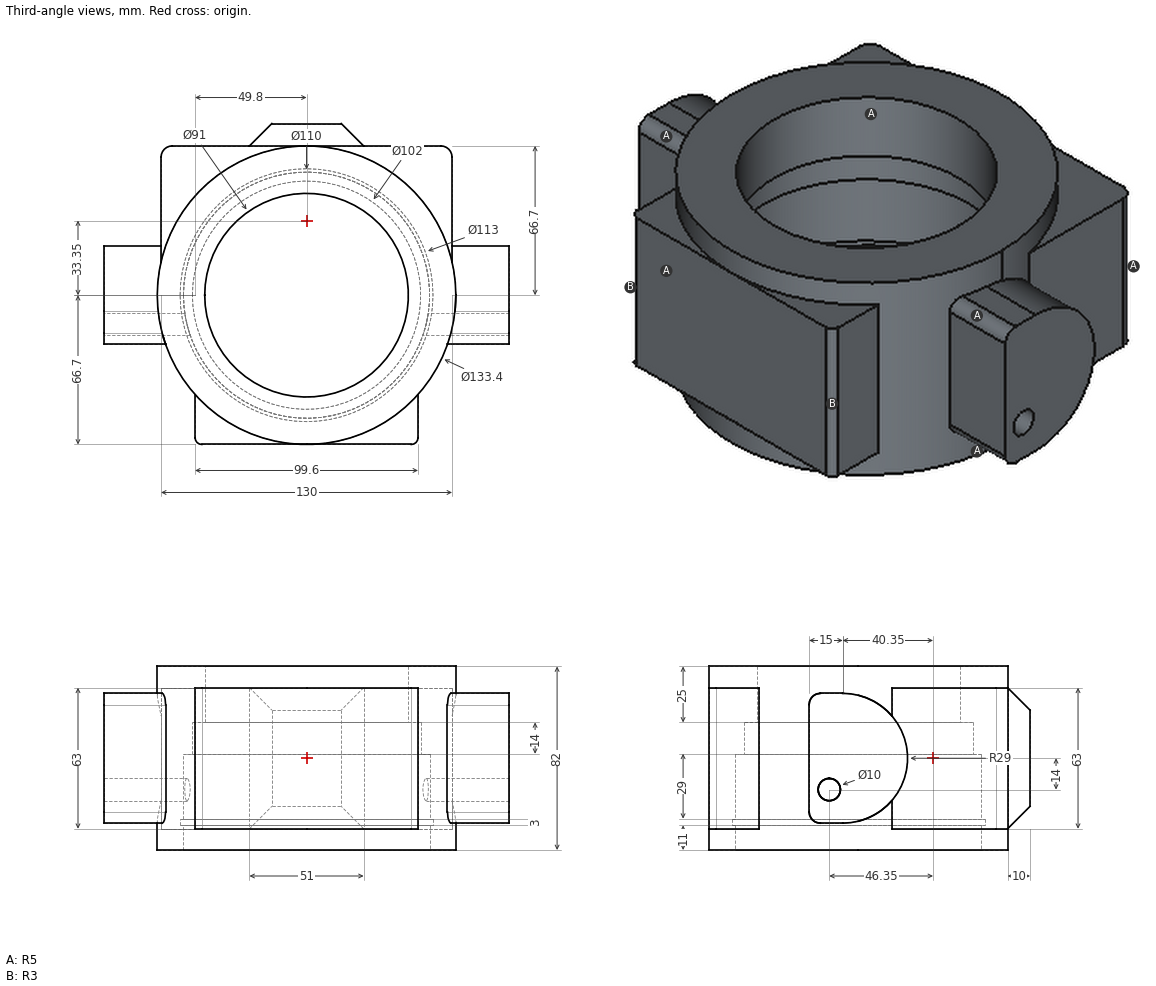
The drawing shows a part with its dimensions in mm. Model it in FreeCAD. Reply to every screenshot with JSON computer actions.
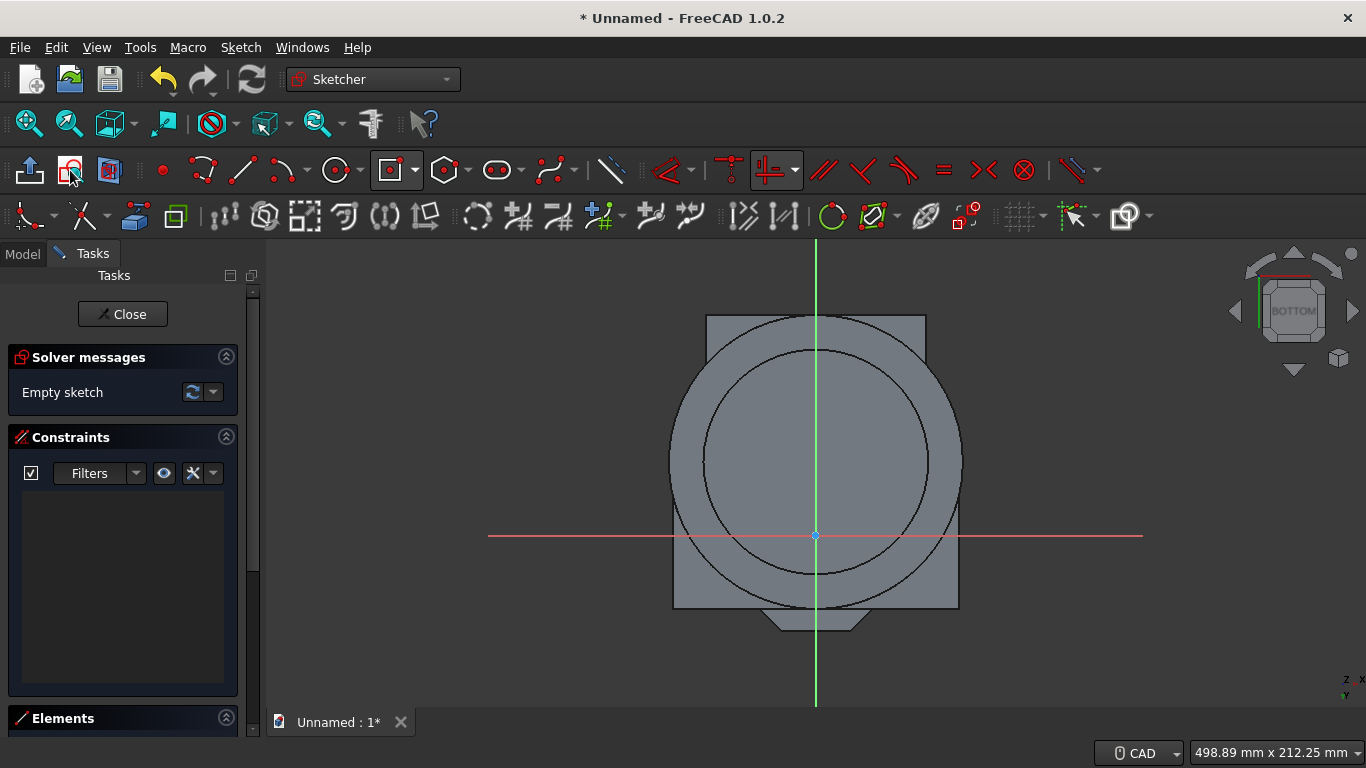
{"action": "scroll", "coordinate": [955, 440], "scroll_direction": "up", "scroll_amount": 2}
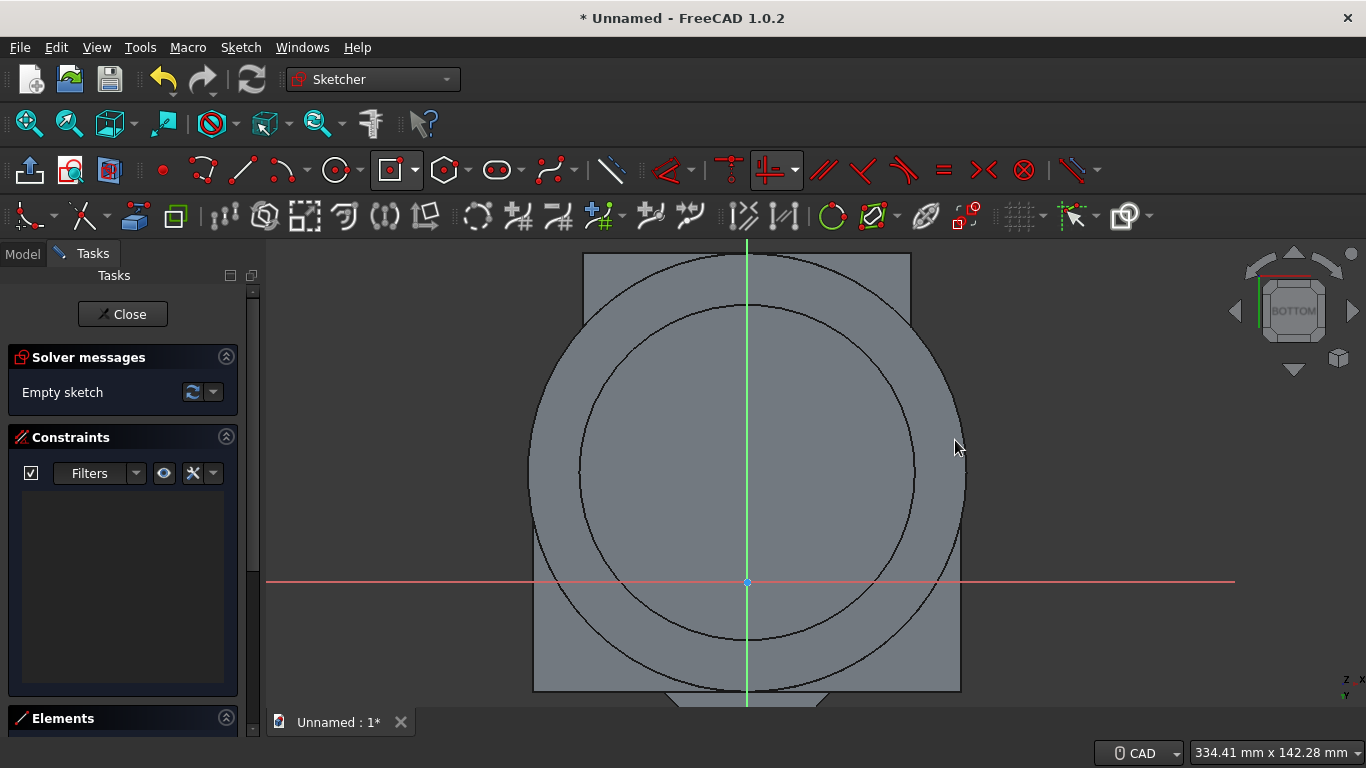
{"action": "left_click", "coordinate": [336, 170]}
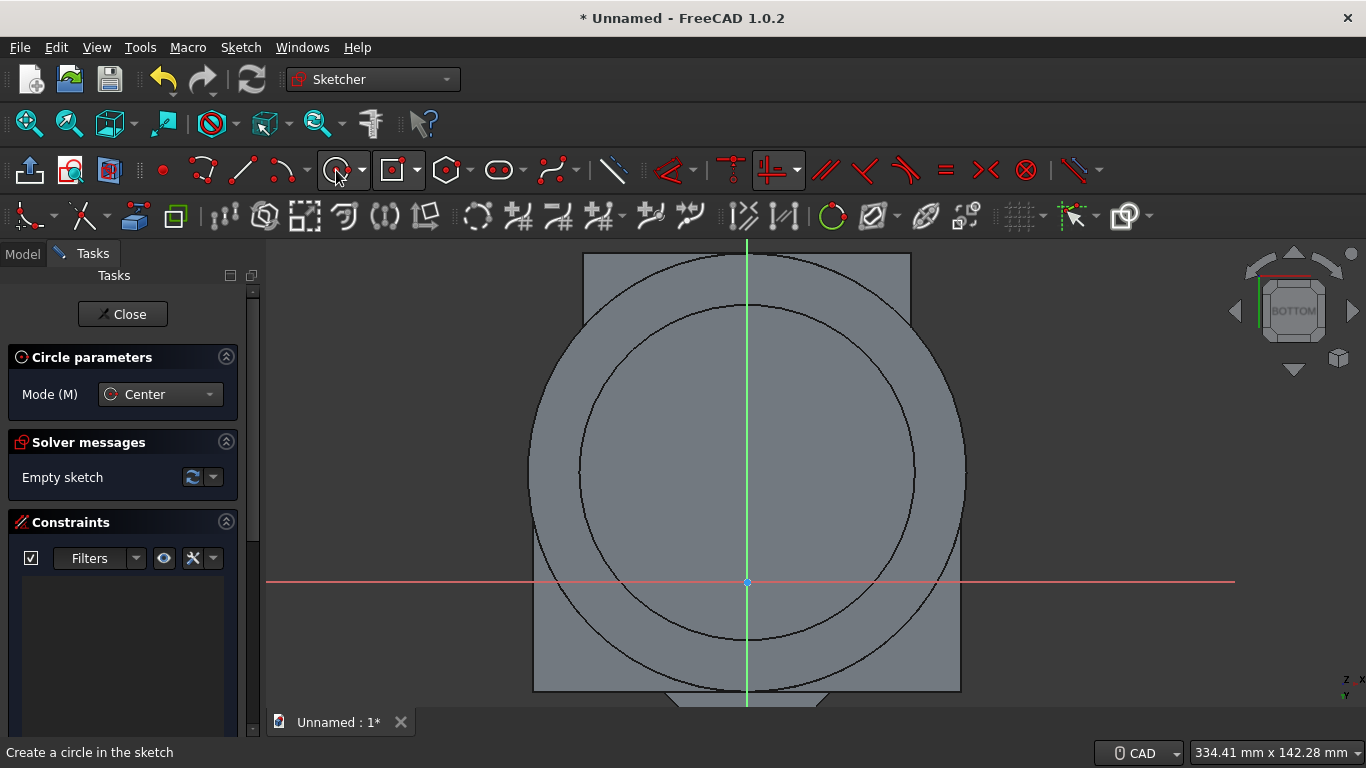
{"action": "left_click", "coordinate": [747, 473]}
{"action": "left_click", "coordinate": [853, 367]}
{"action": "key", "text": "Escape"}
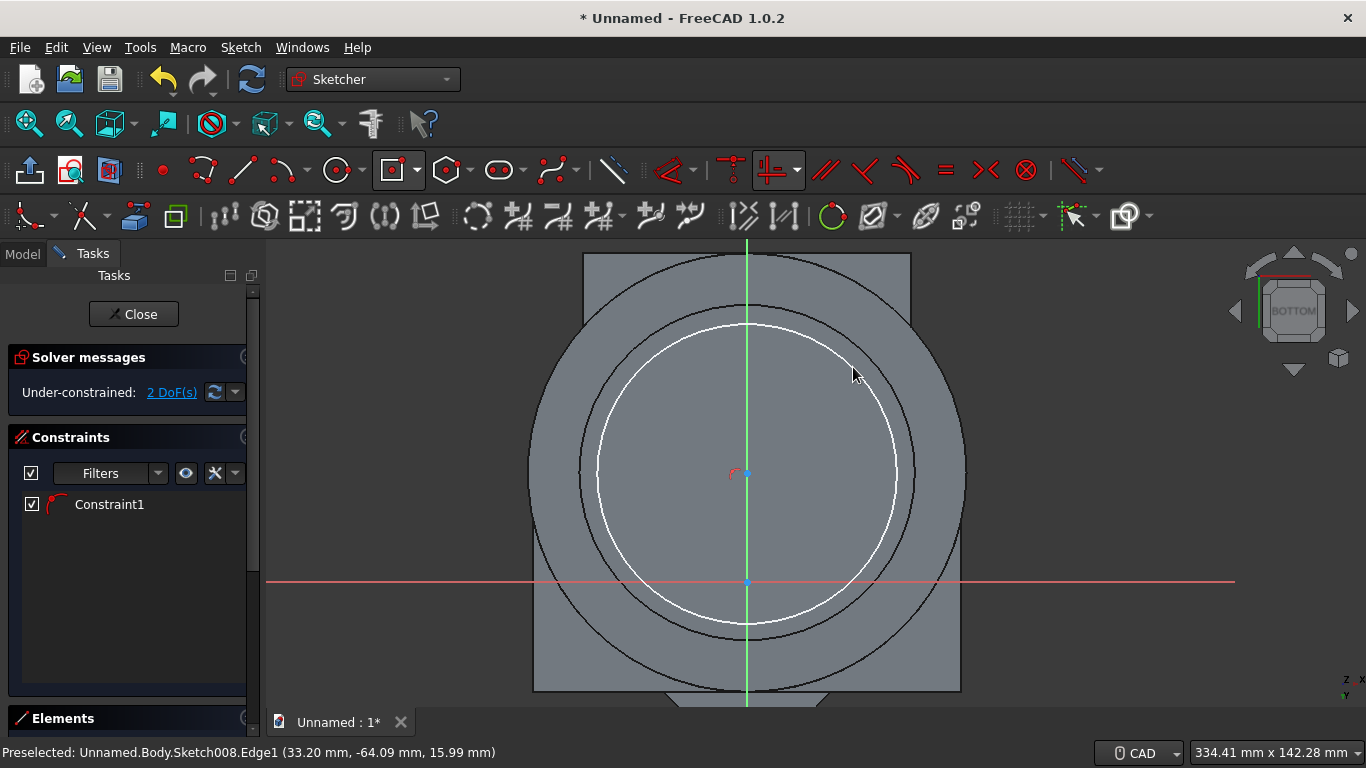
{"action": "left_click", "coordinate": [668, 170]}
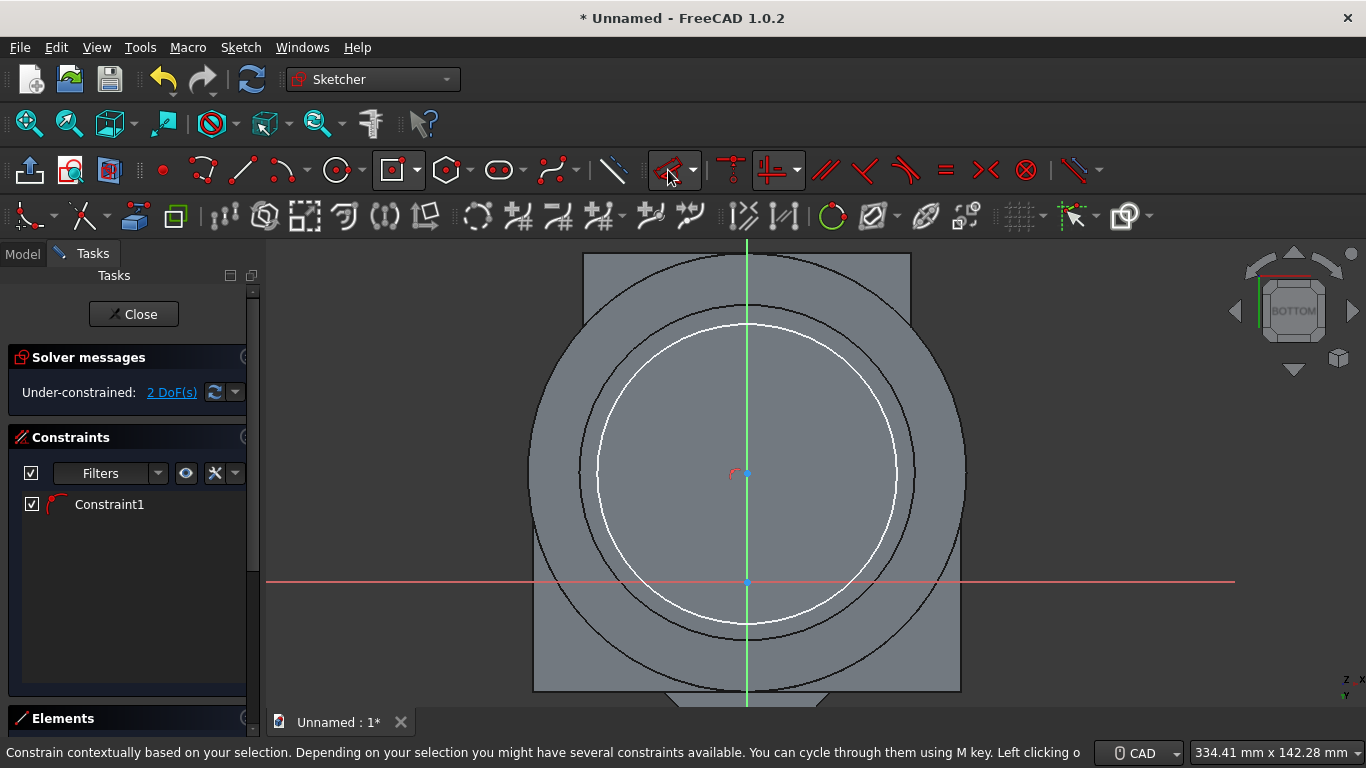
{"action": "left_click", "coordinate": [853, 368]}
{"action": "left_click", "coordinate": [876, 345]}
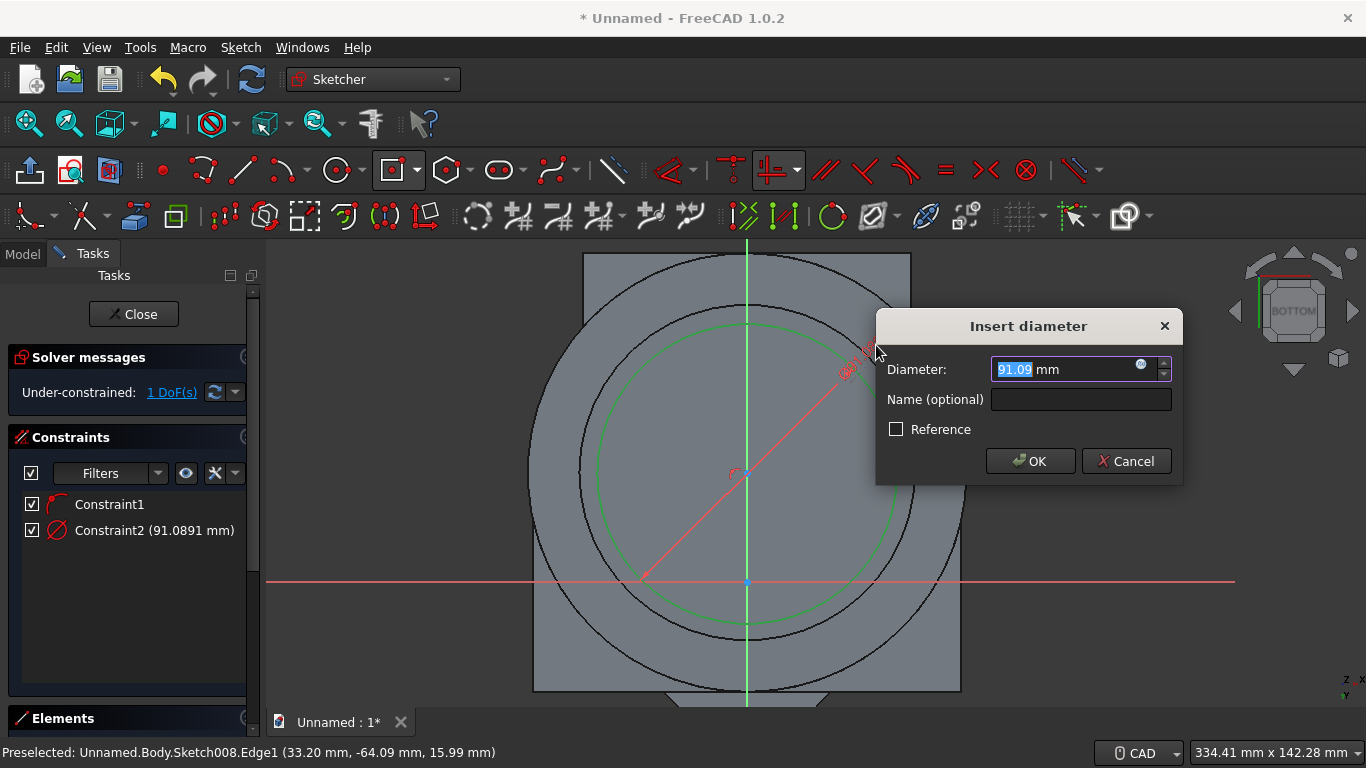
{"action": "type", "text": "91"}
{"action": "key", "text": "Return"}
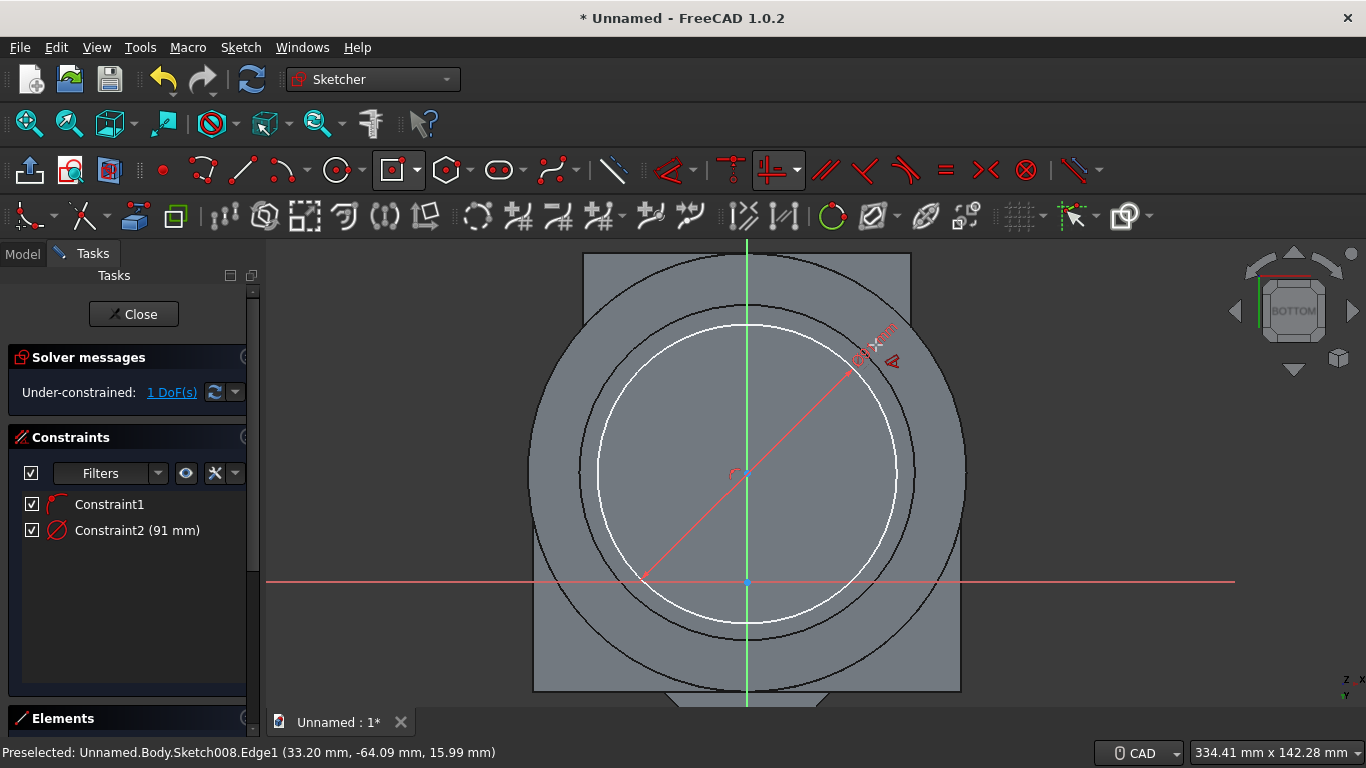
{"action": "left_click", "coordinate": [747, 474]}
{"action": "left_click", "coordinate": [781, 528]}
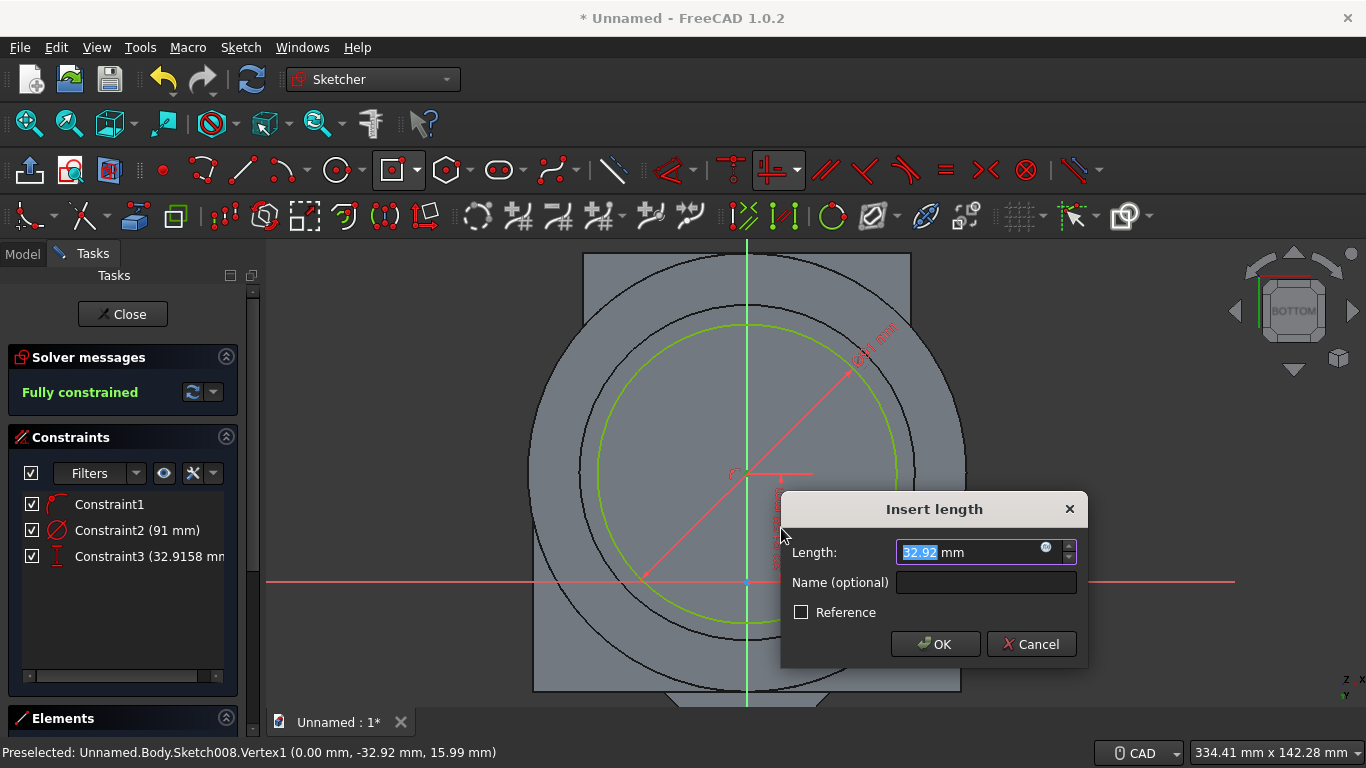
{"action": "type", "text": "33.35"}
{"action": "key", "text": "Return"}
{"action": "key", "text": "Escape"}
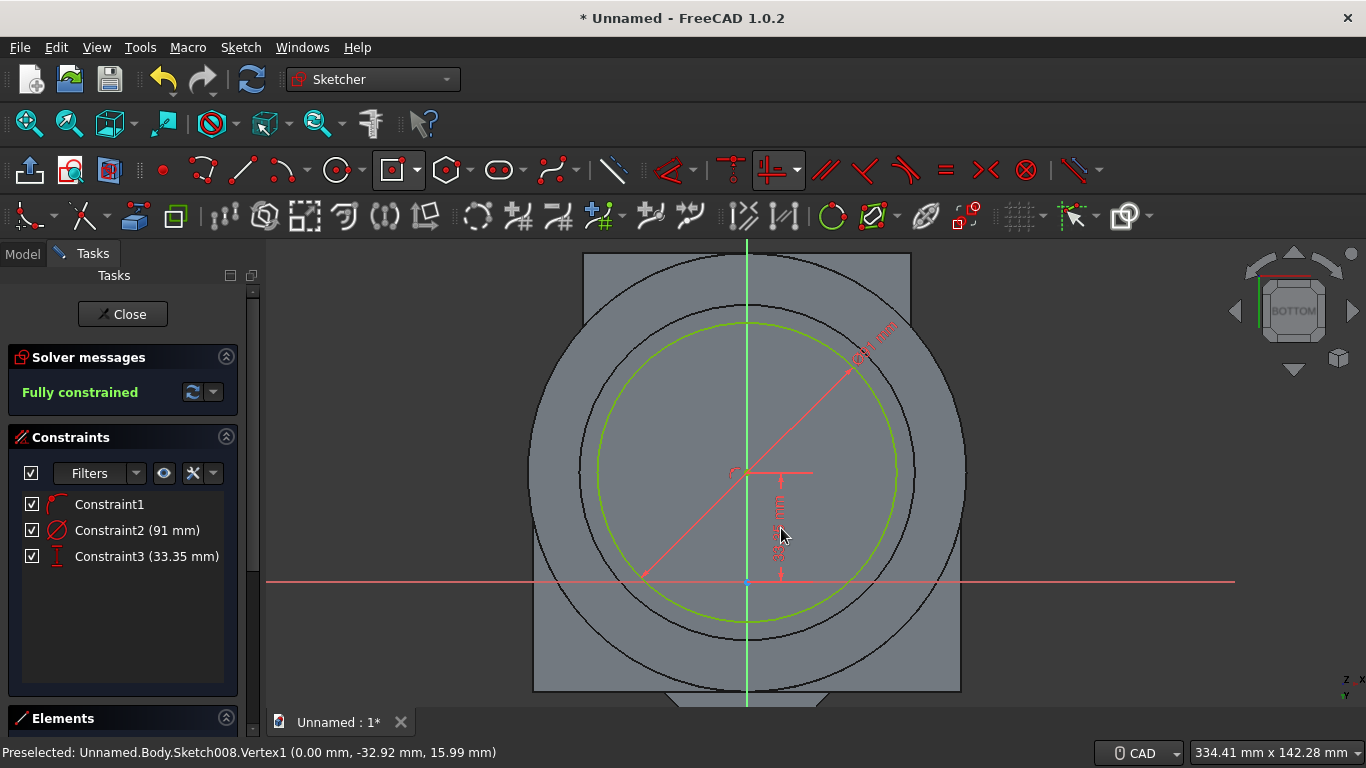
{"action": "left_click", "coordinate": [123, 314]}